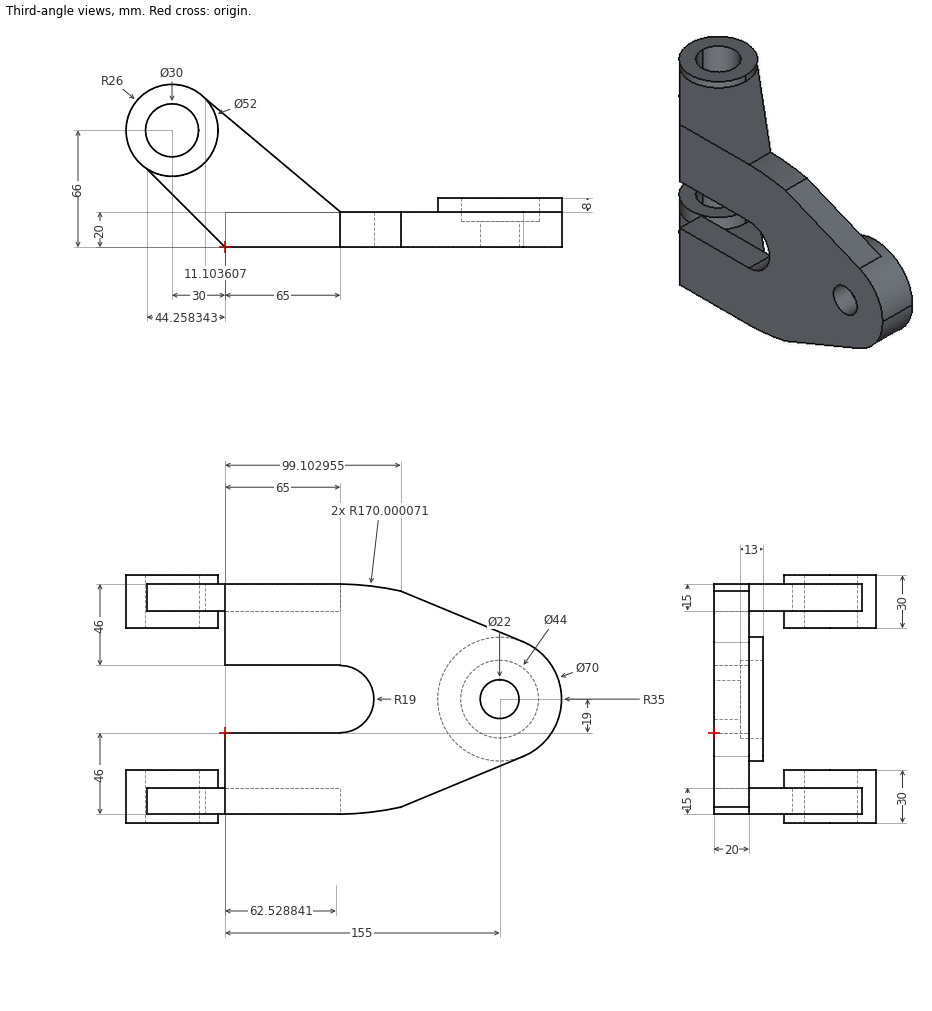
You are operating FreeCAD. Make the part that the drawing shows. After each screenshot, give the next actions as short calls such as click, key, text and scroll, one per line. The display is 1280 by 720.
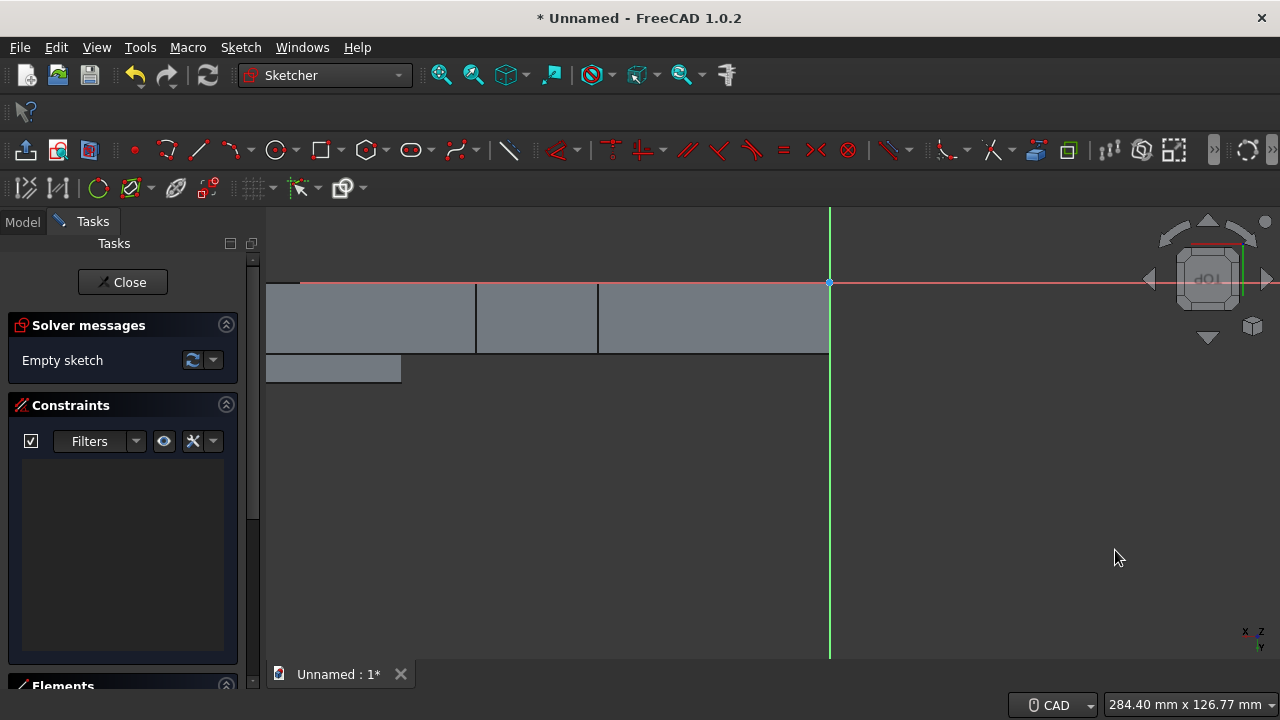
click(168, 150)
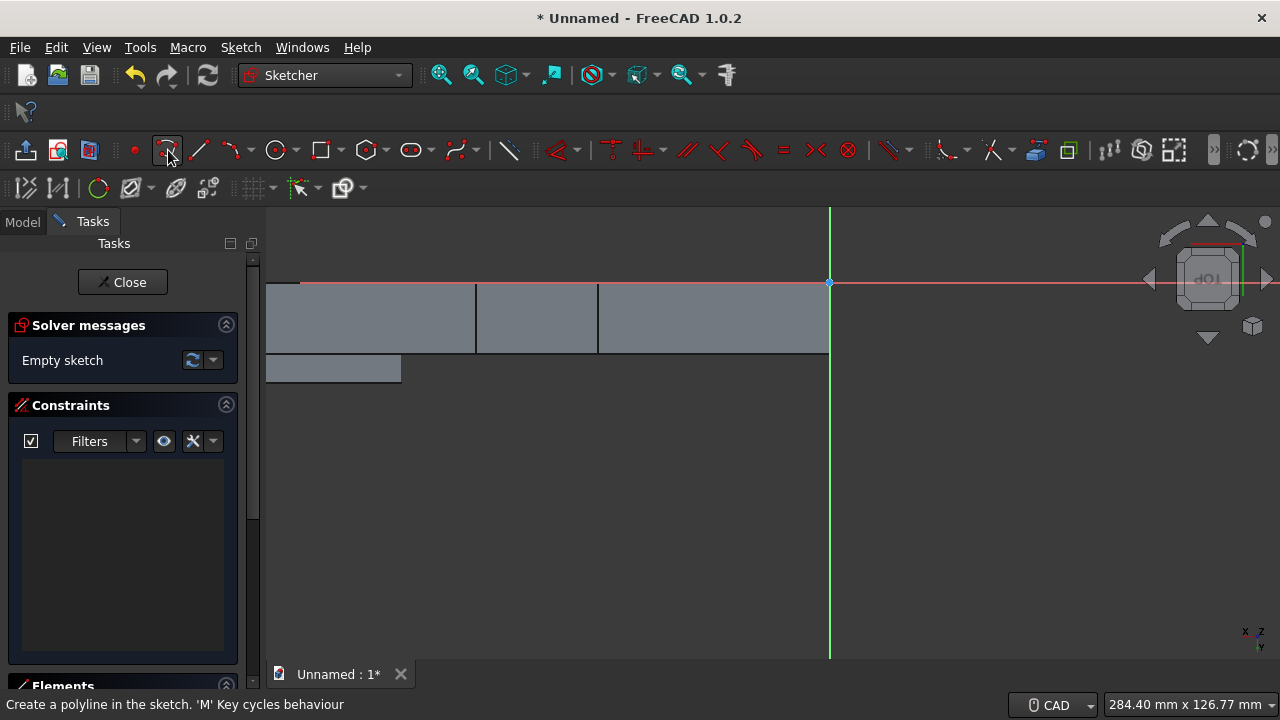
click(987, 441)
click(830, 283)
click(598, 292)
click(598, 354)
click(869, 582)
right_click(869, 582)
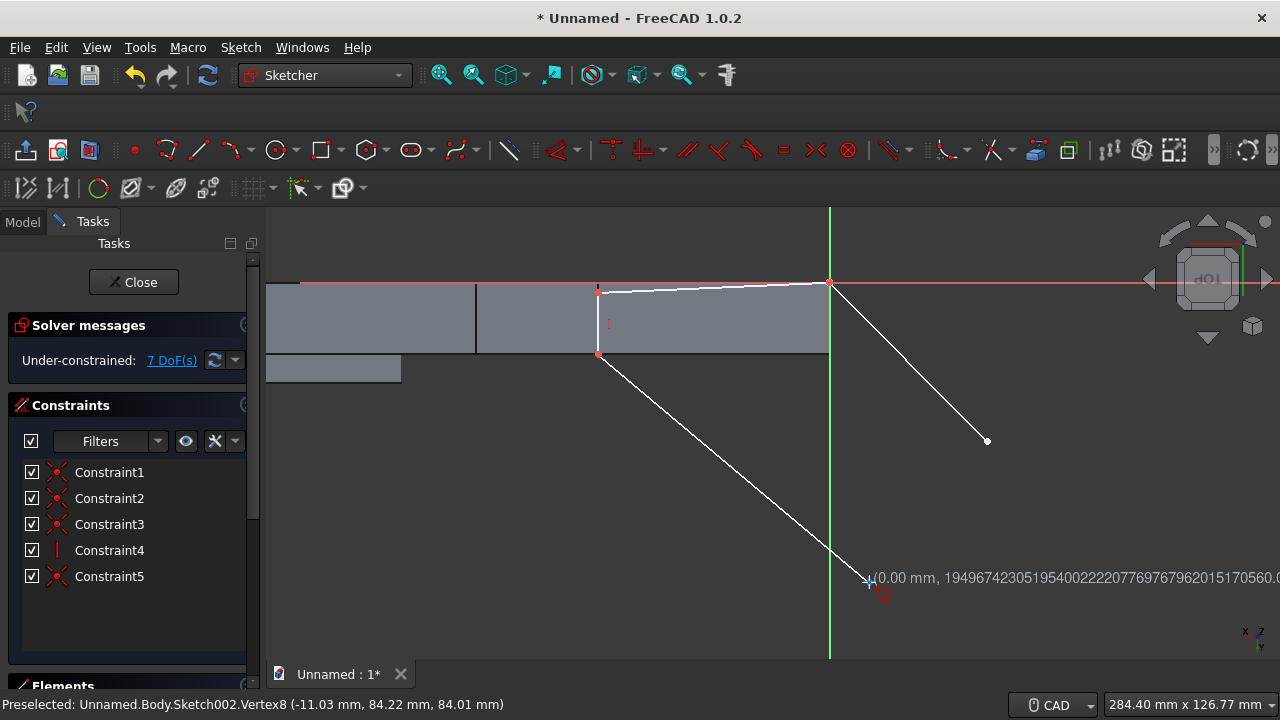
key(g)
key(3)
key(a)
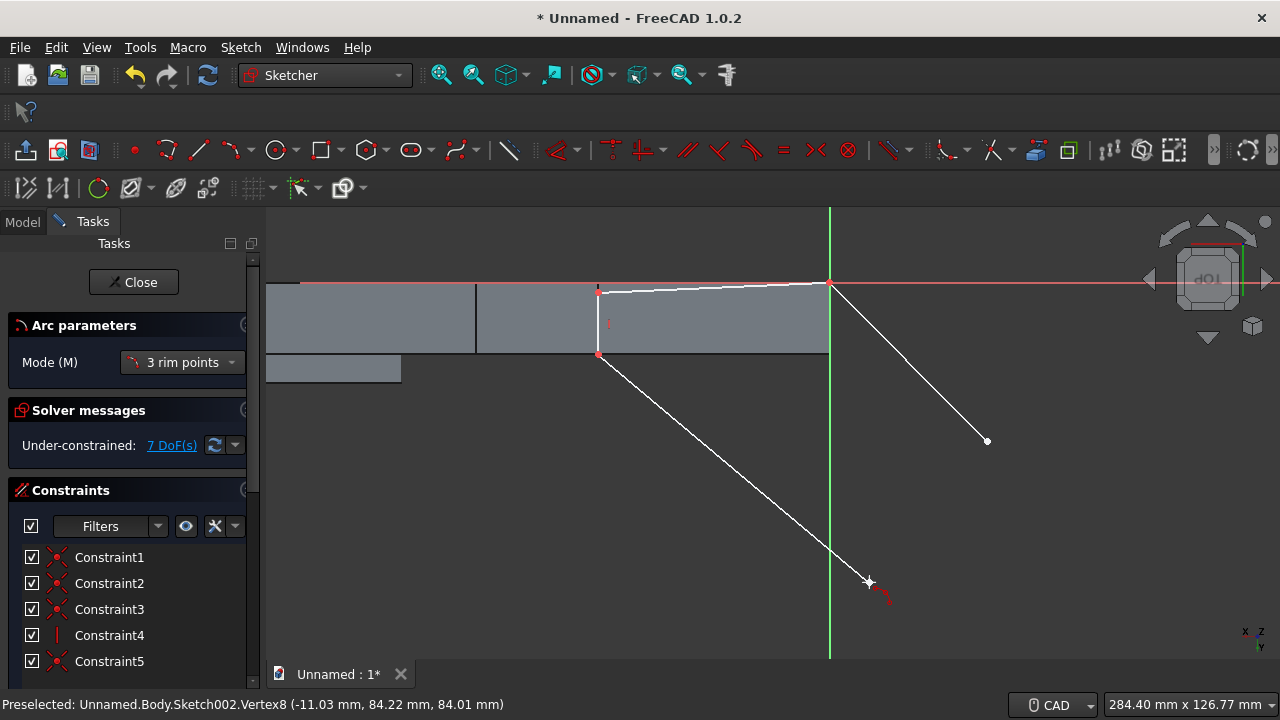
click(869, 583)
click(987, 442)
click(1008, 578)
key(Escape)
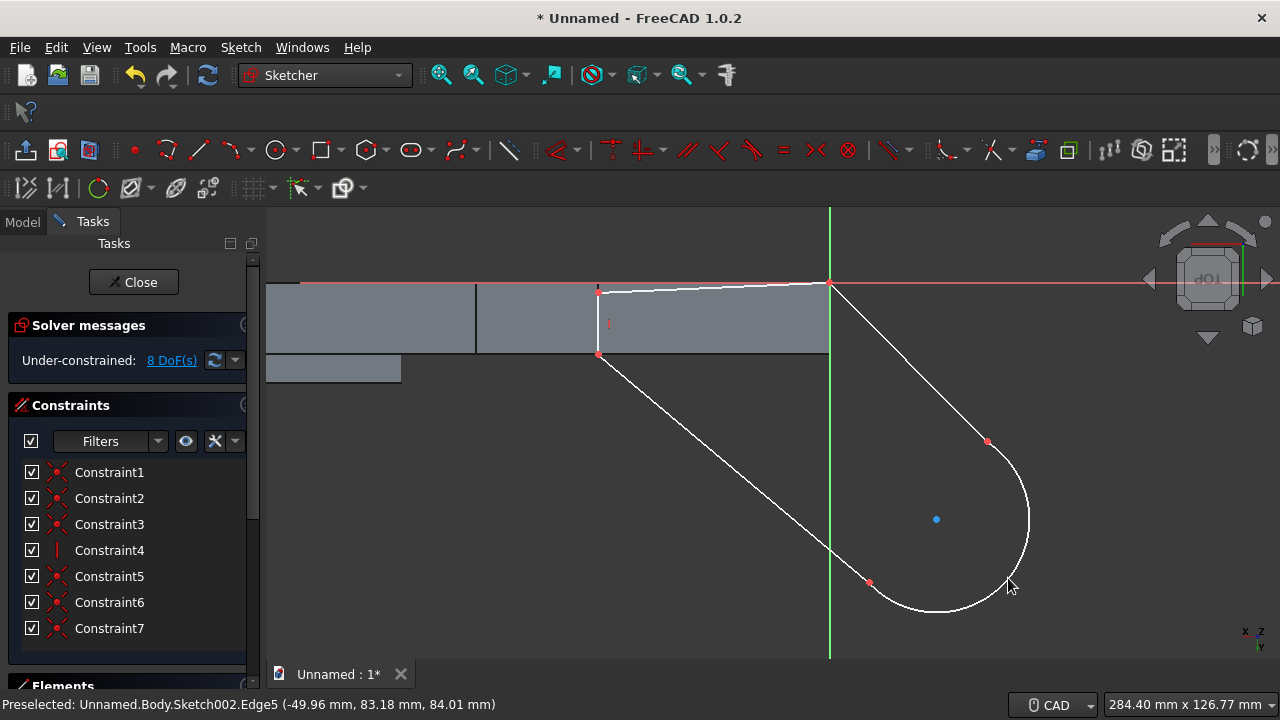
click(760, 286)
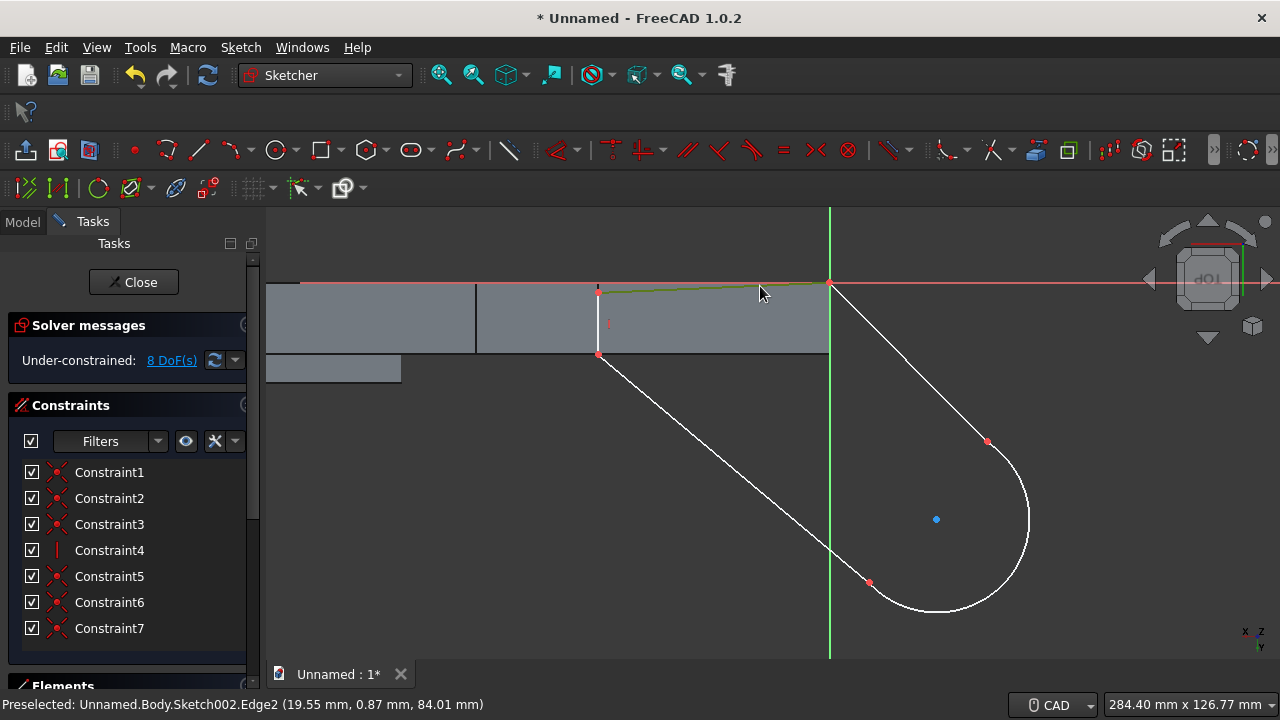
key(h)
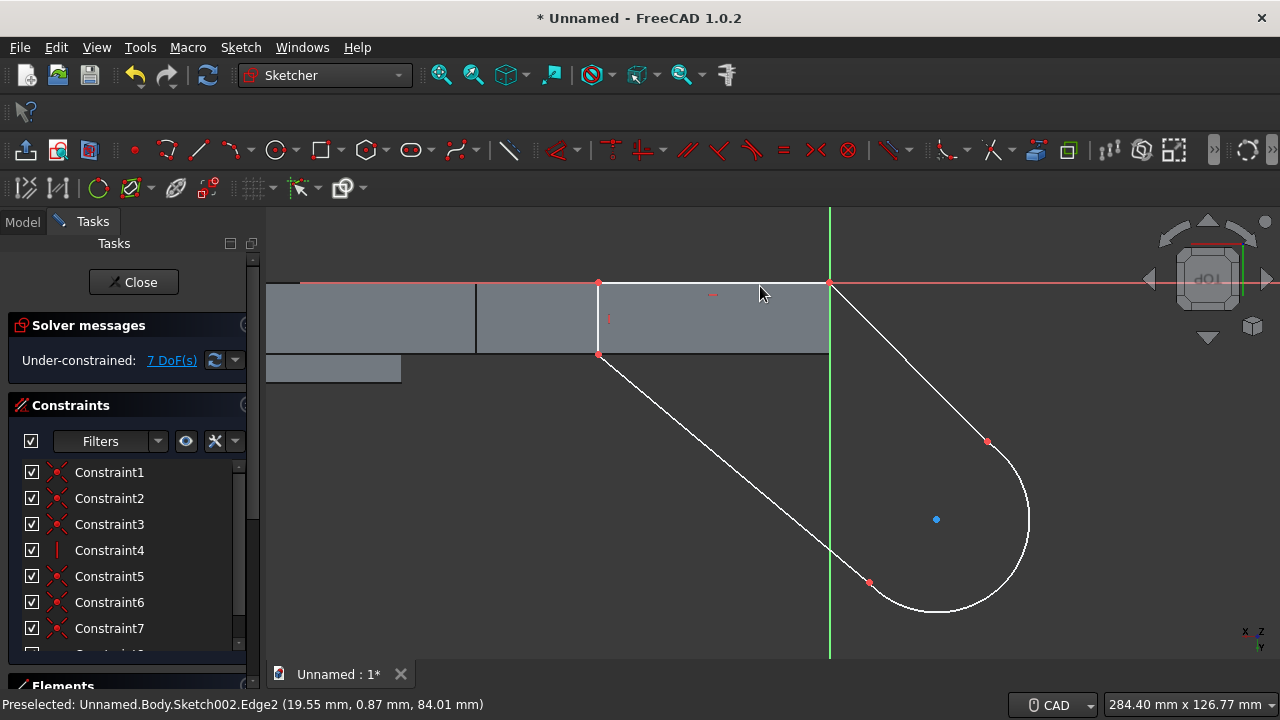
key(d)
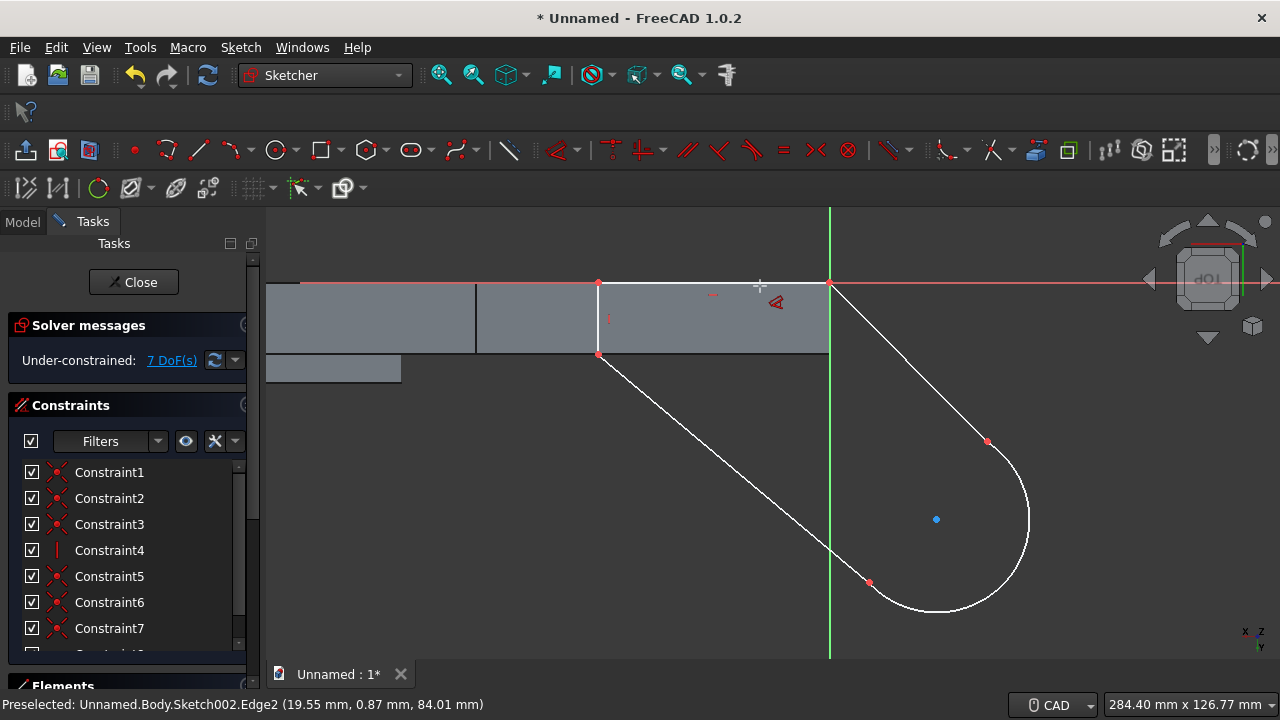
click(955, 611)
click(1017, 616)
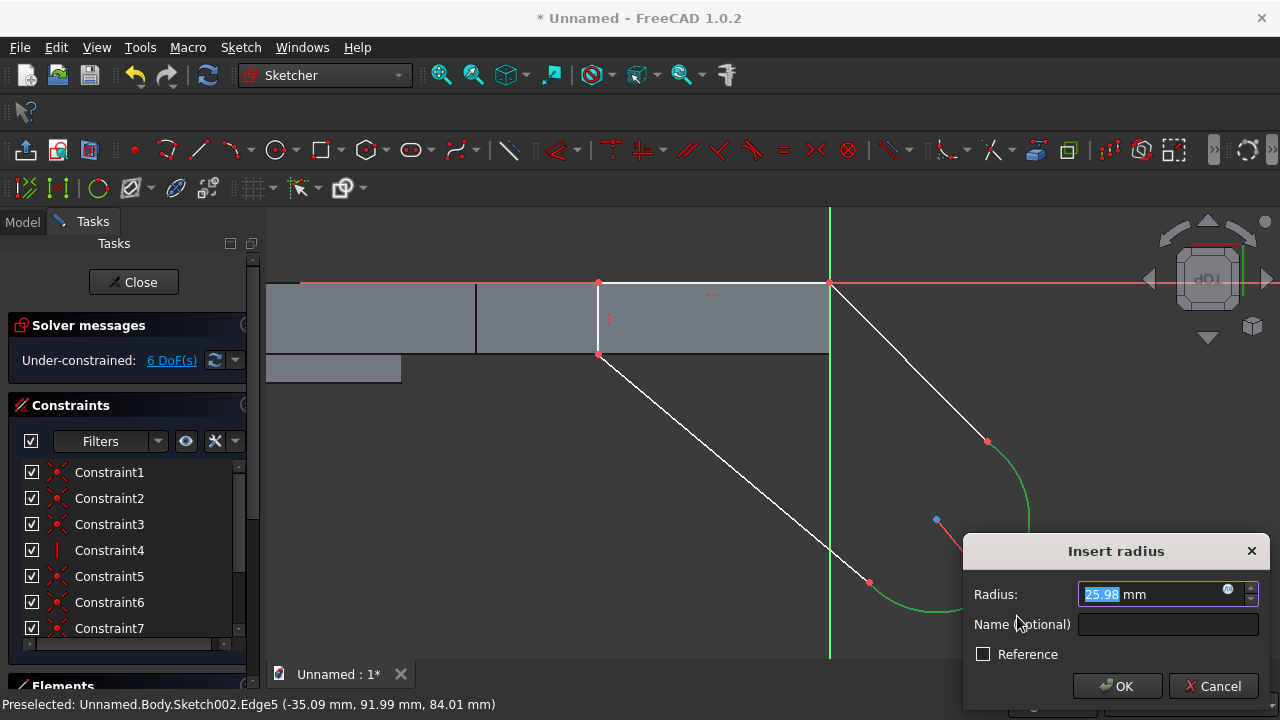
text(26)
key(Return)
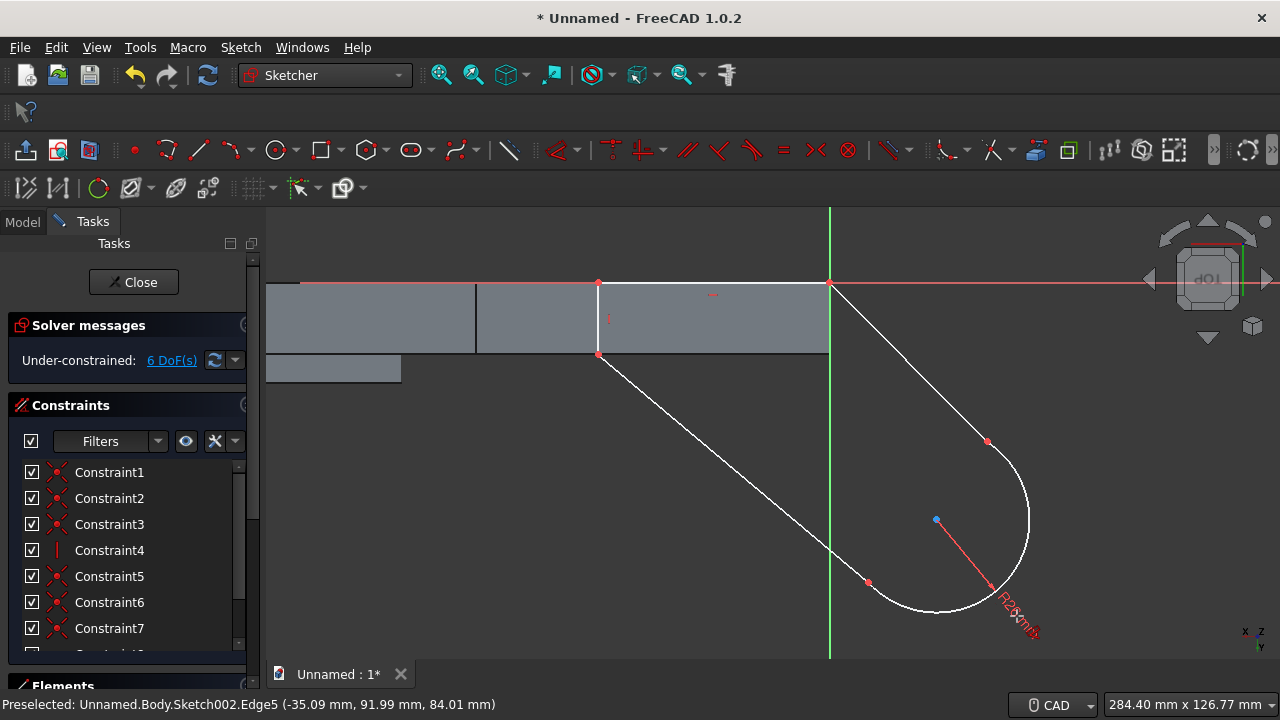
click(760, 283)
click(714, 249)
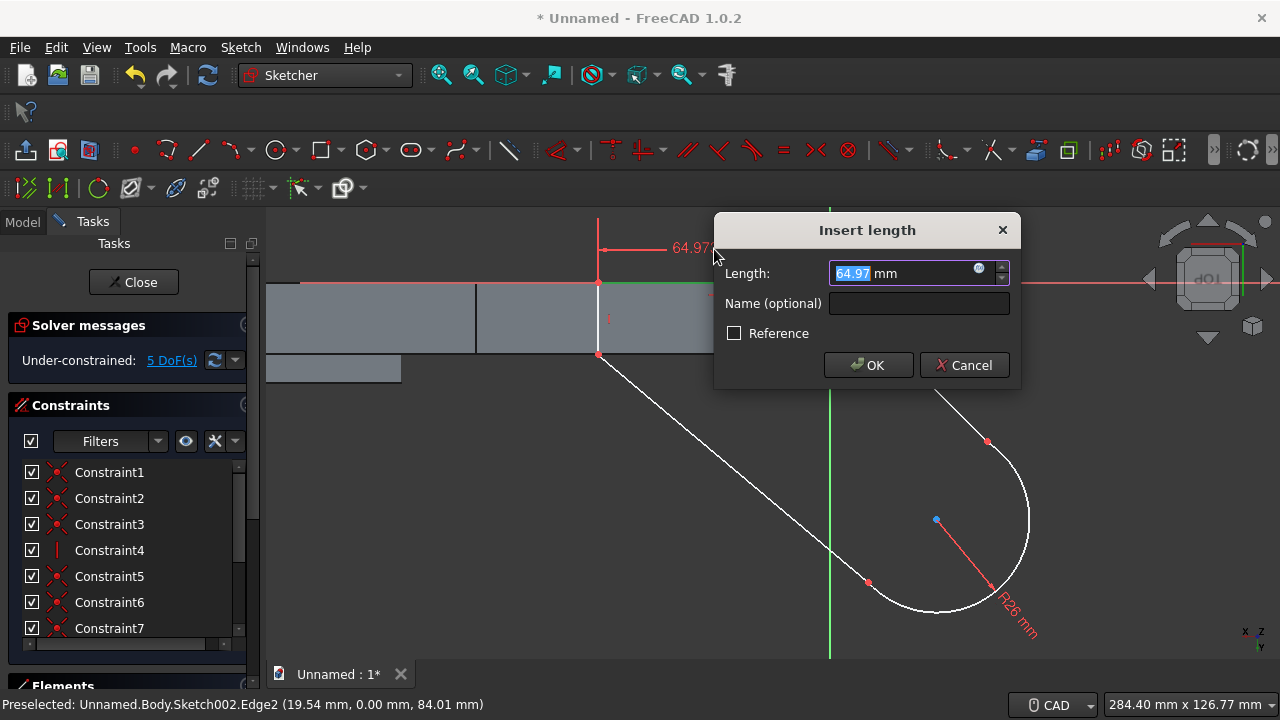
text(65)
key(Return)